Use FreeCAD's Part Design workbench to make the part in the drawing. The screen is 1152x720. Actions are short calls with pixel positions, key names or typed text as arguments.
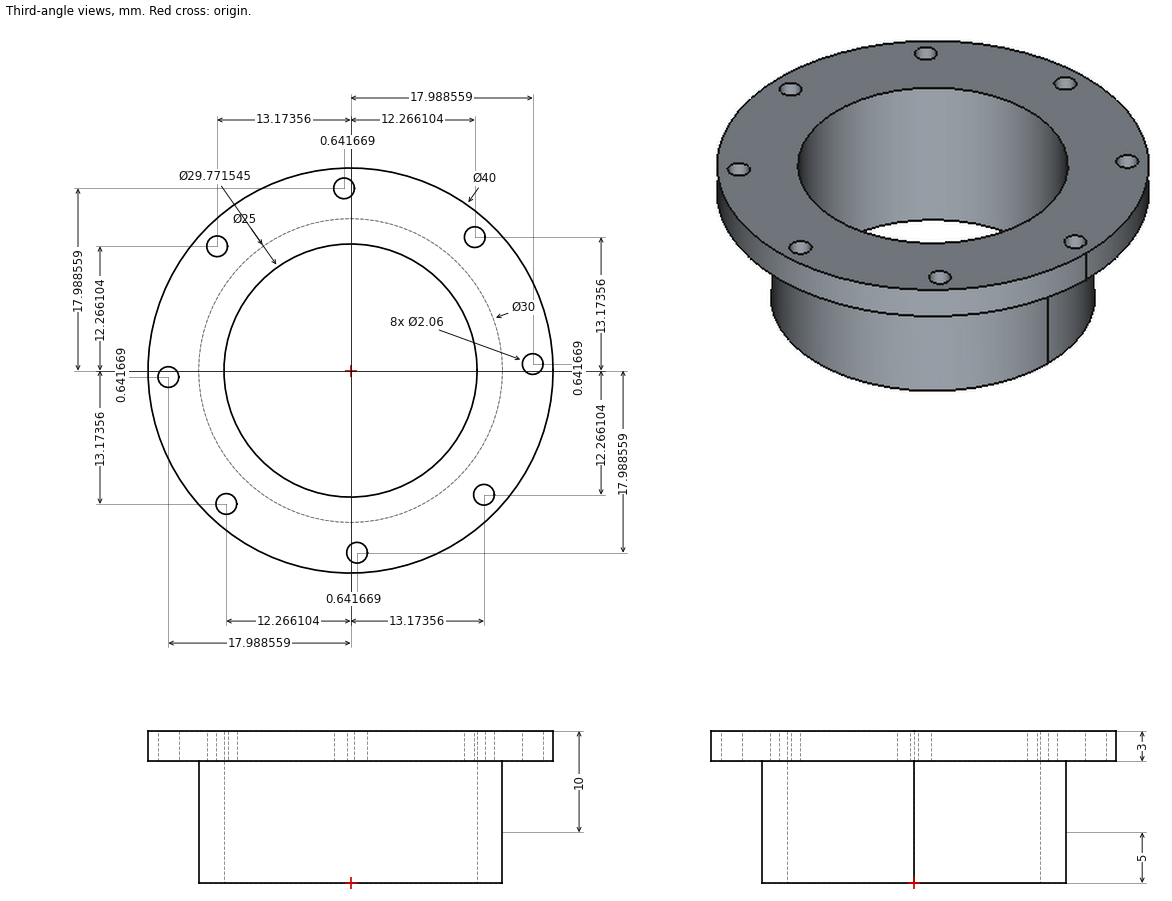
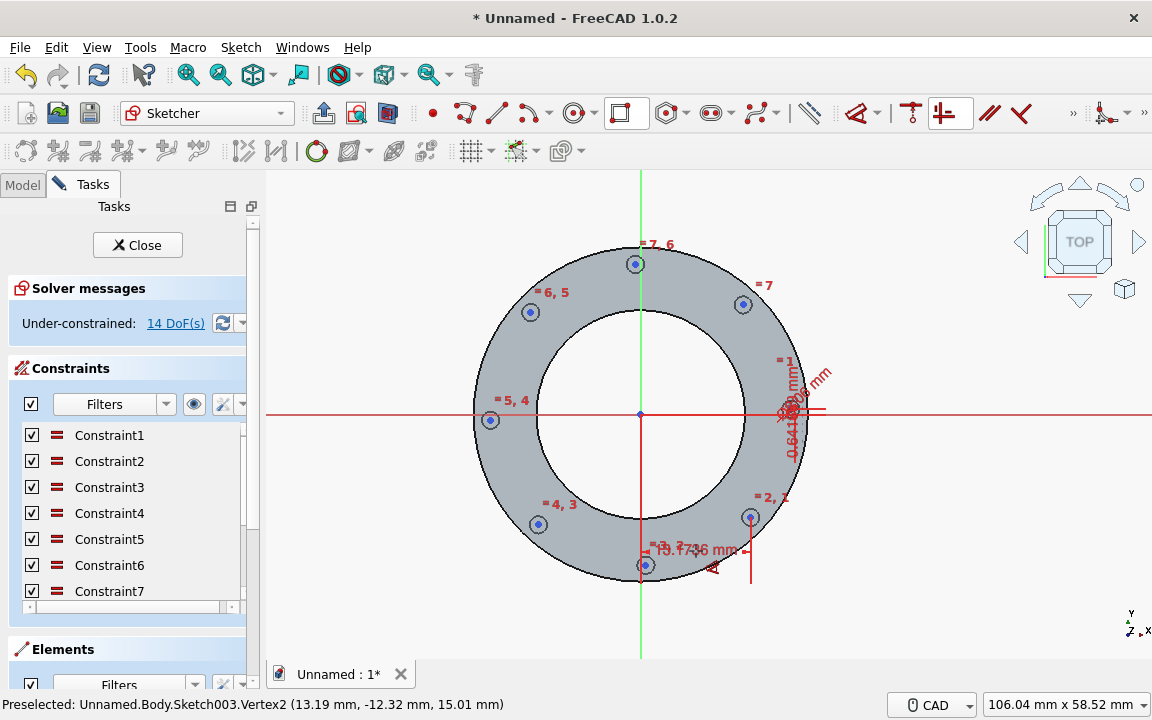
scroll(646, 565, up, 11)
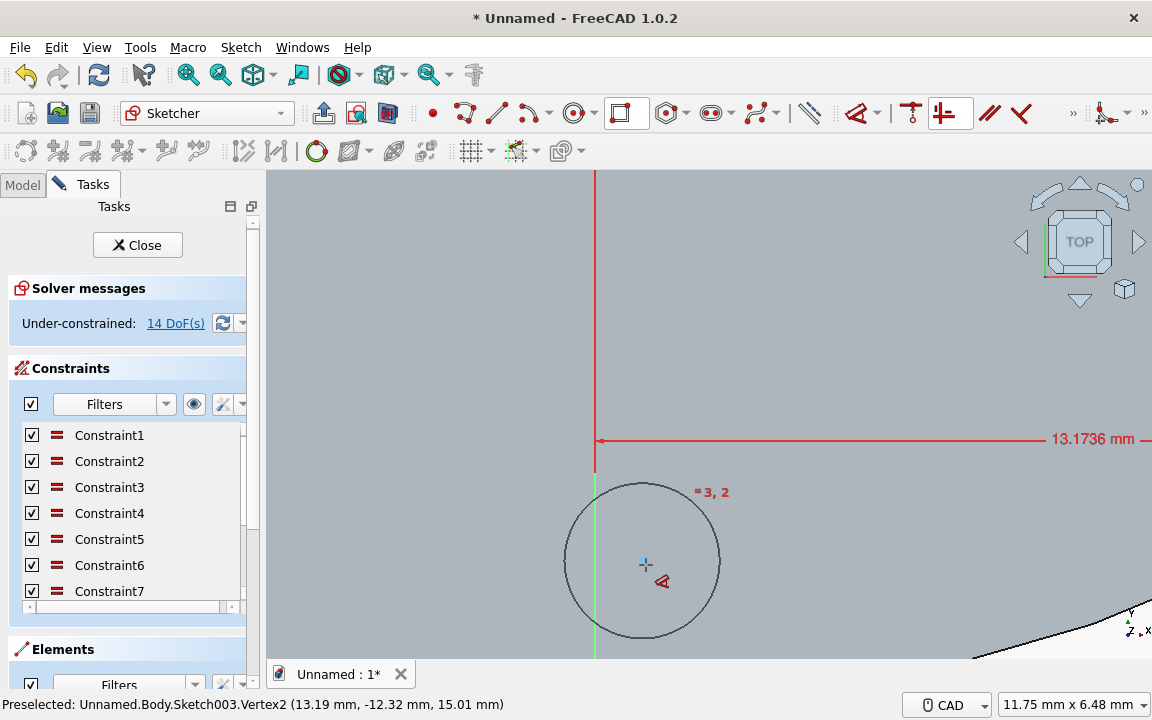
click(642, 561)
click(618, 595)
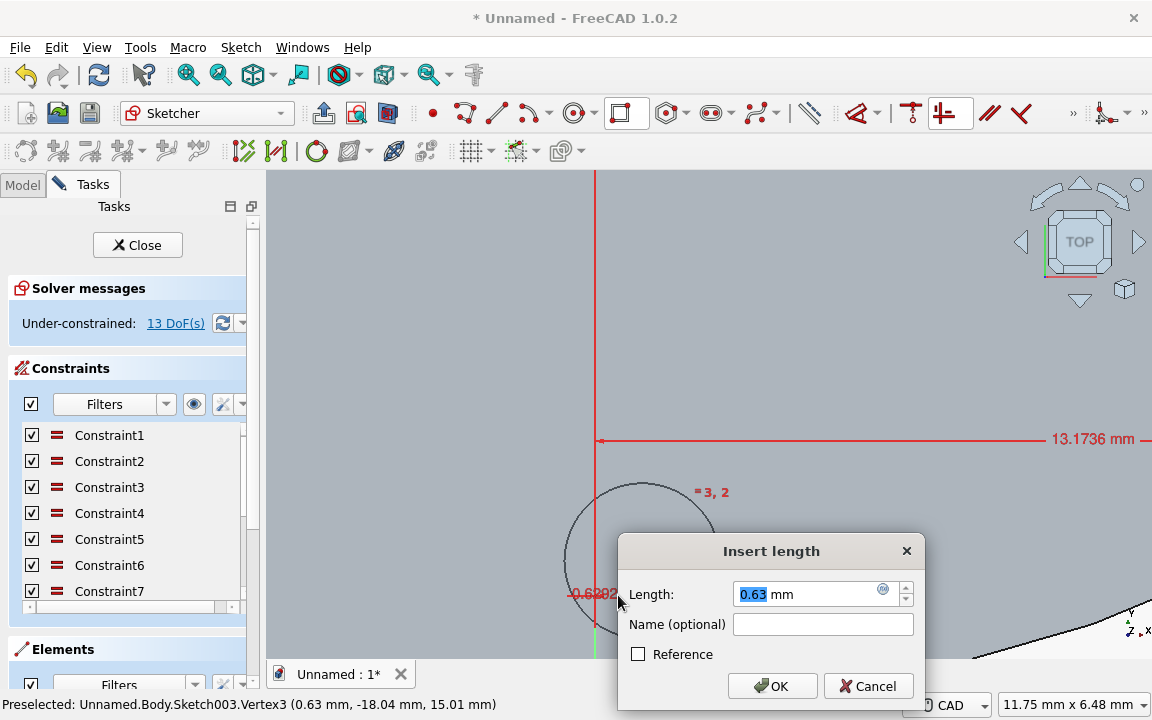
text(0.641669)
key(Return)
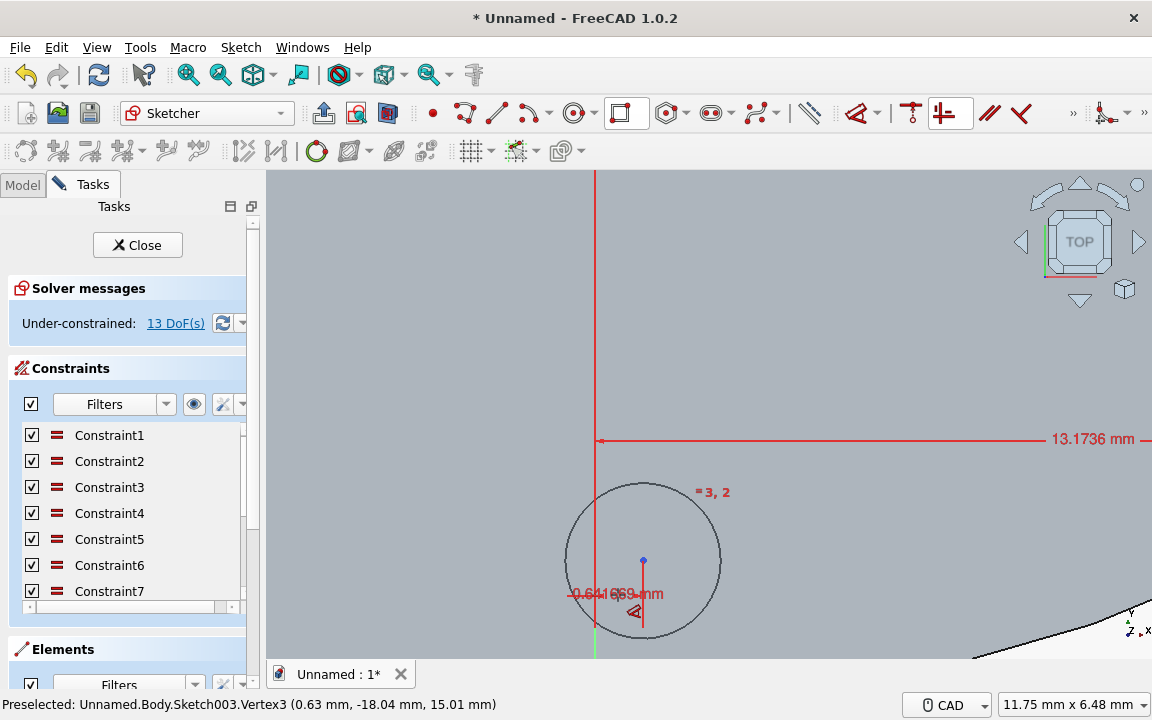
scroll(646, 566, down, 11)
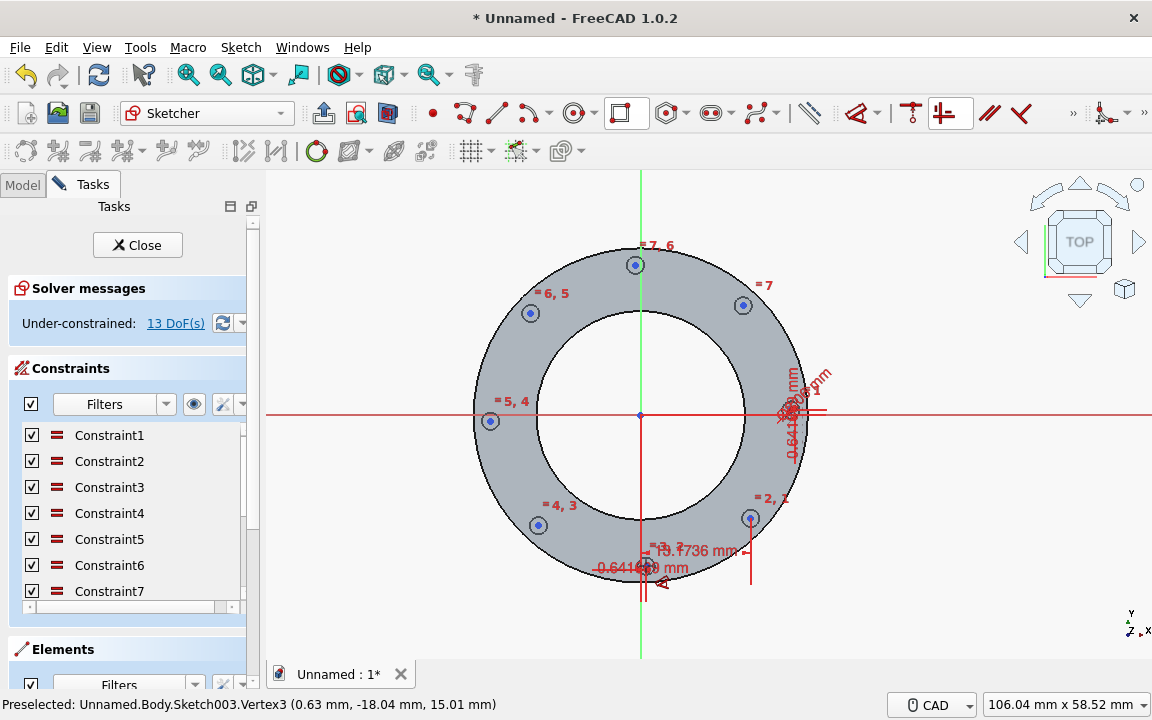
click(538, 526)
click(504, 471)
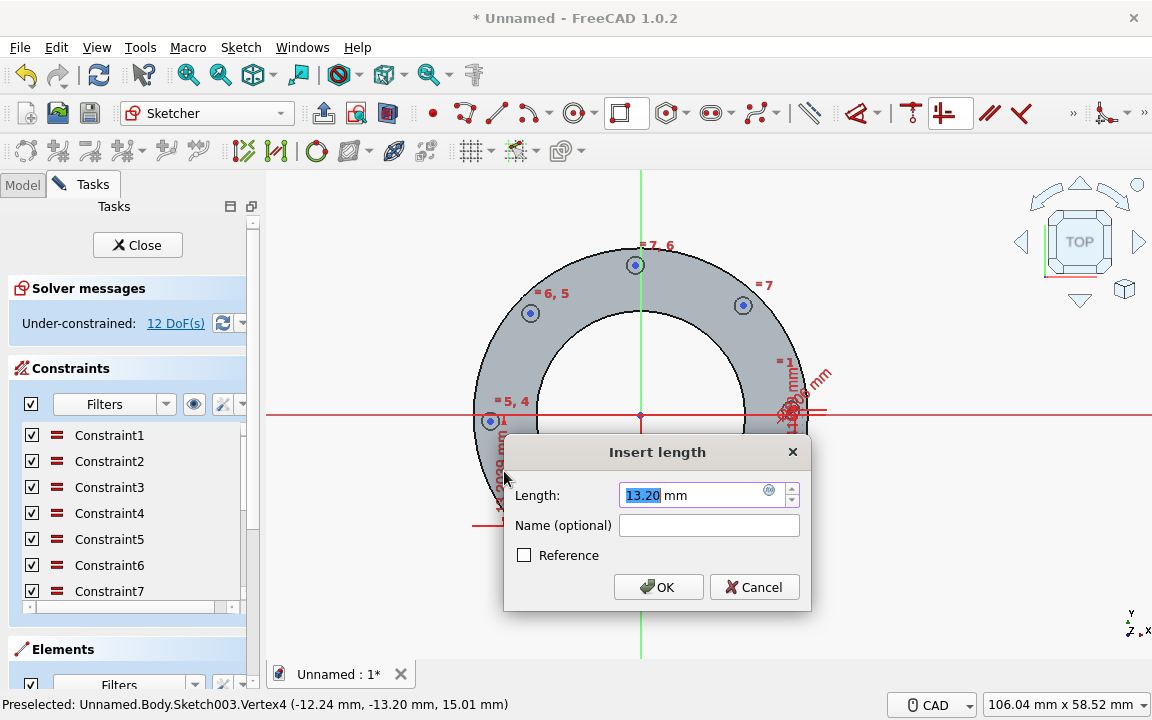
text(13.17356)
key(Return)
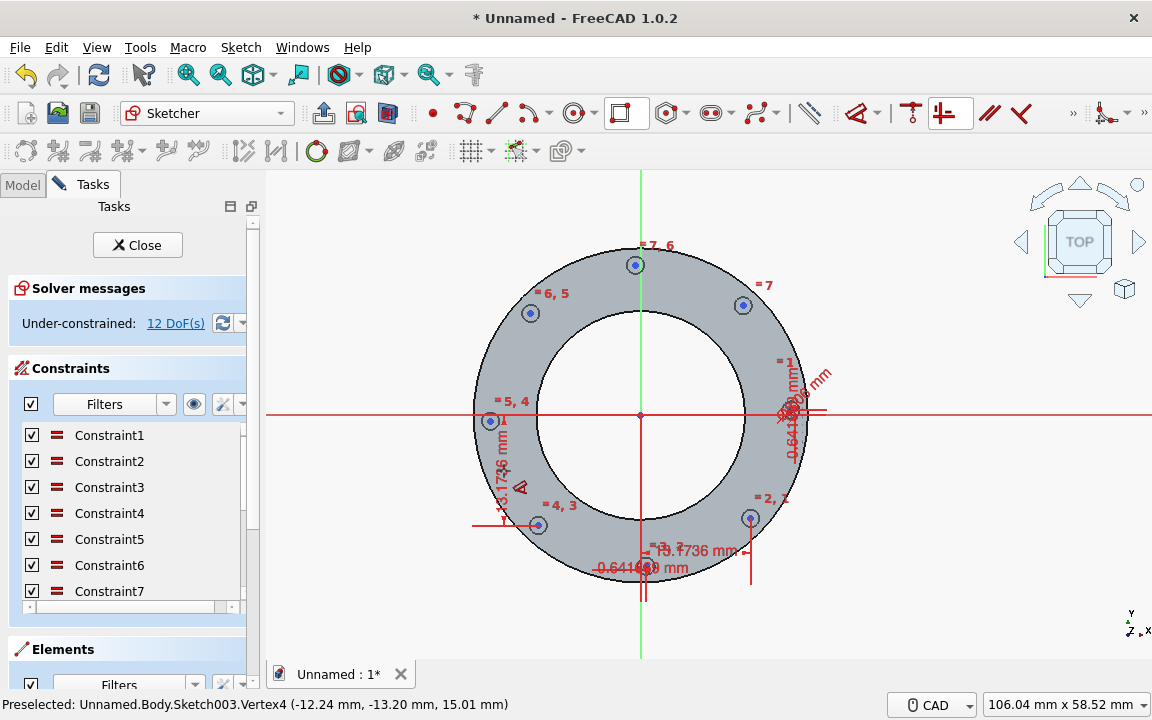
scroll(491, 421, up, 11)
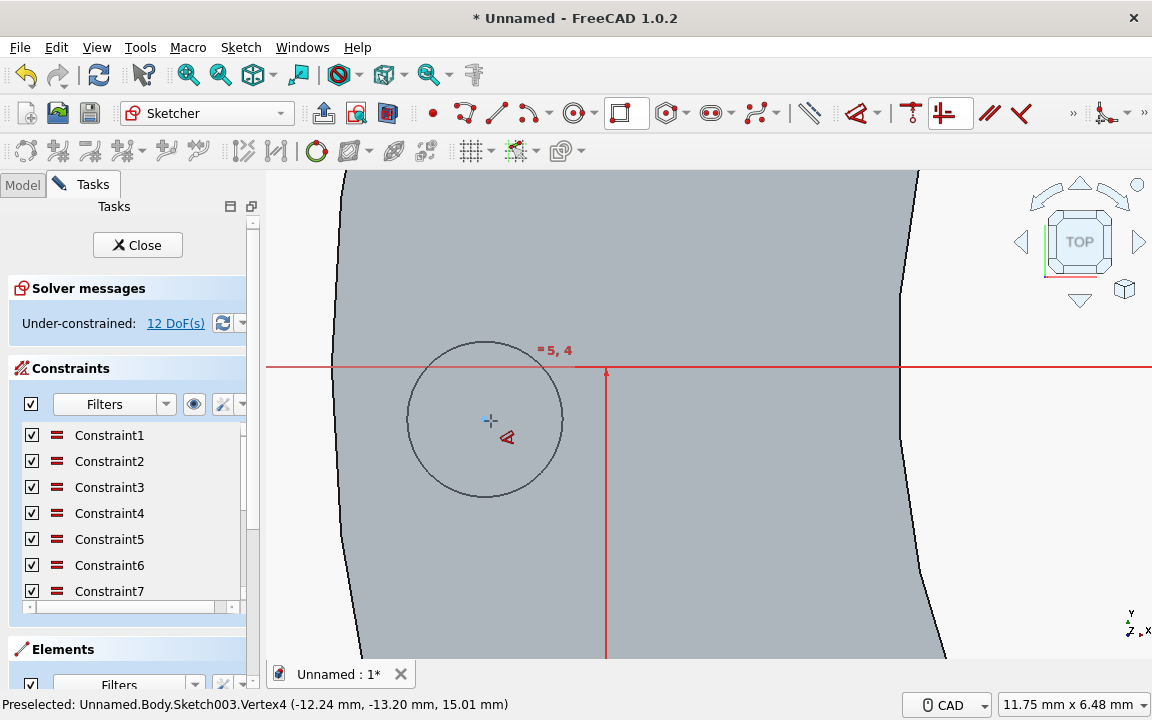
click(485, 419)
click(451, 393)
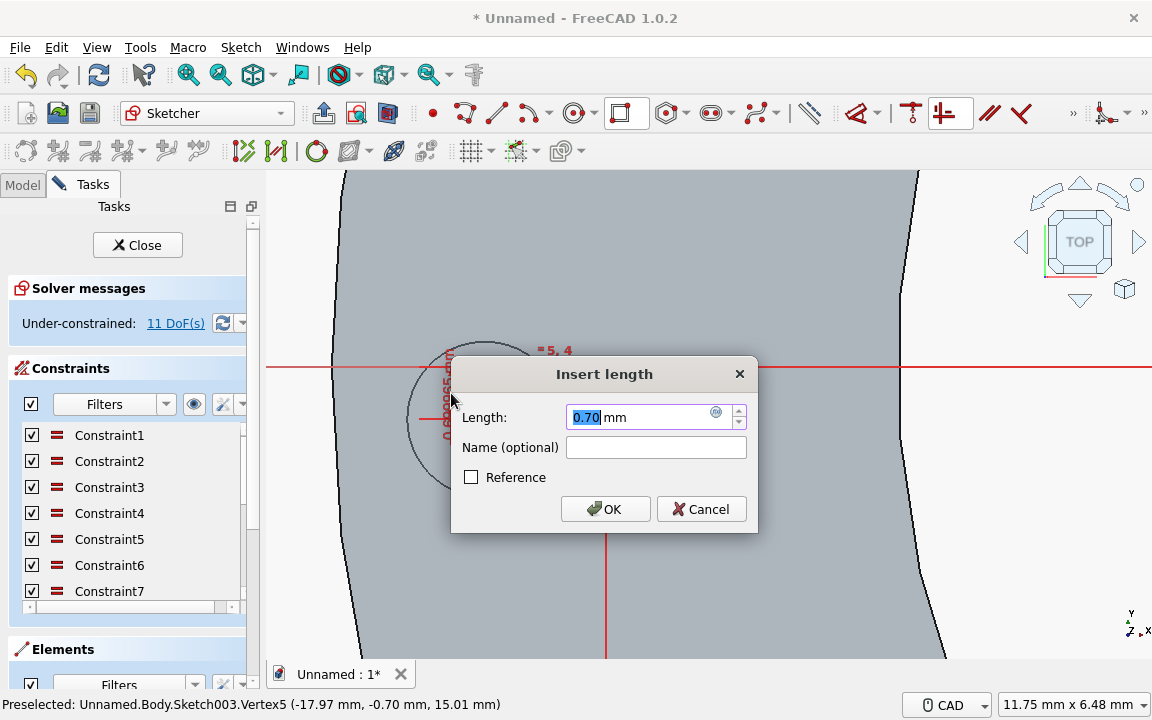
text(0.641669)
key(Return)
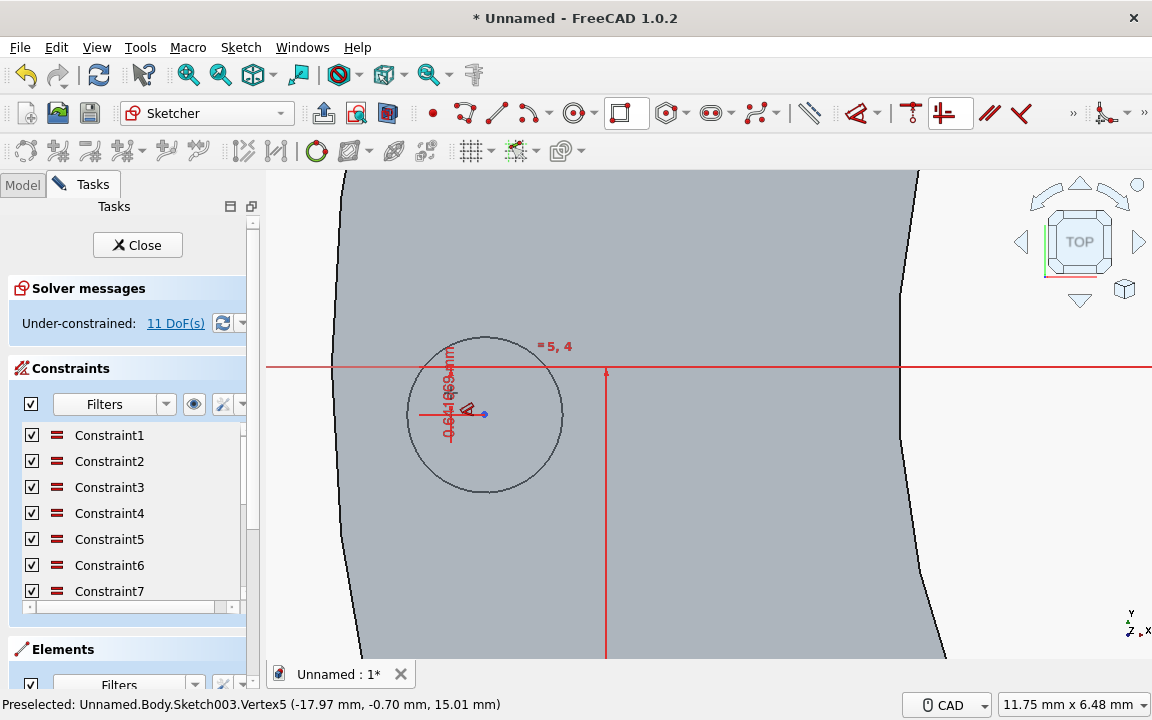
scroll(491, 420, down, 11)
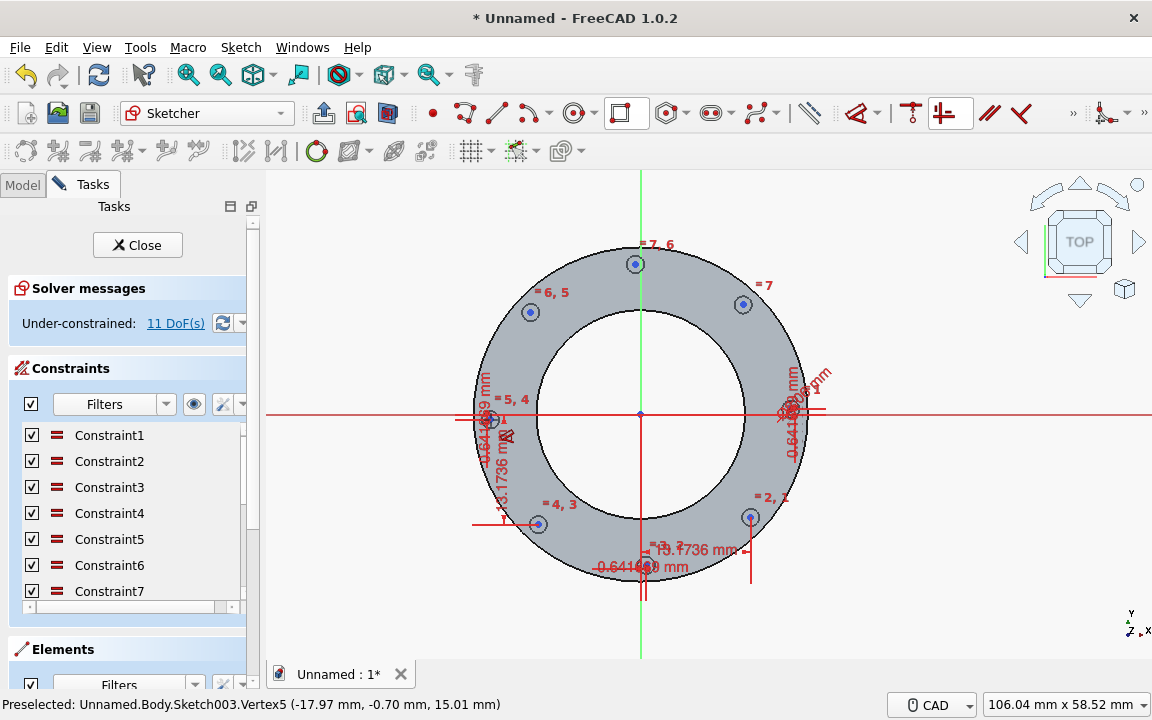
click(531, 313)
click(586, 279)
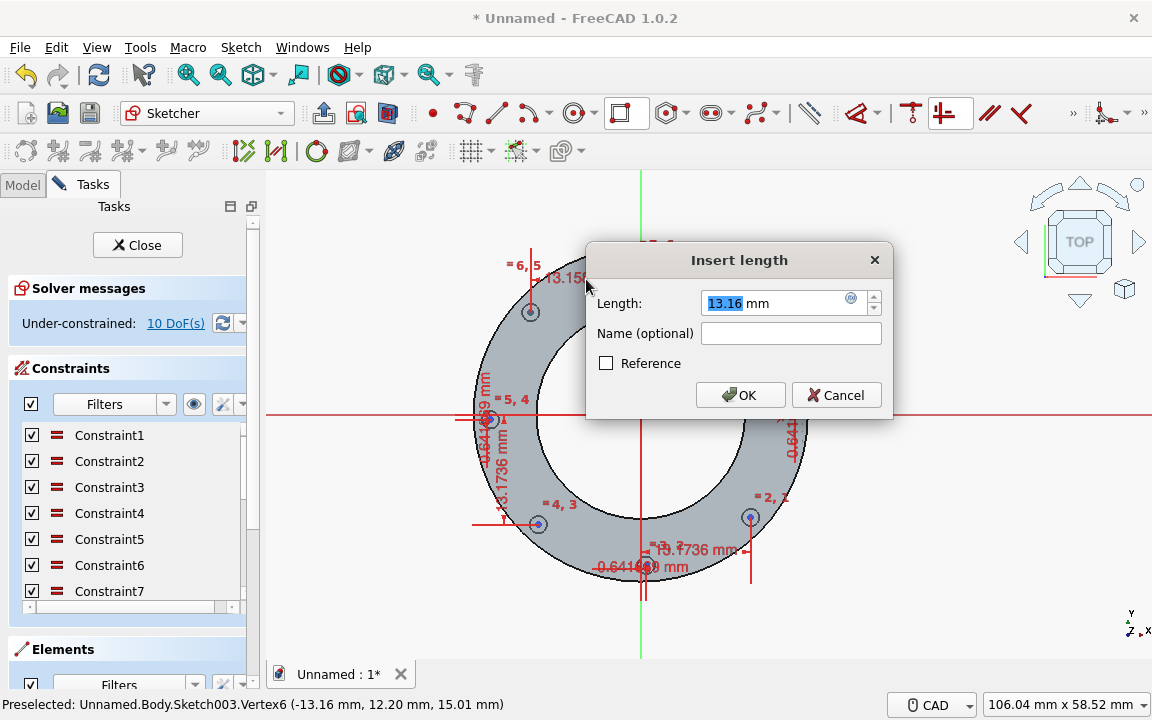
text(13.17356)
key(Return)